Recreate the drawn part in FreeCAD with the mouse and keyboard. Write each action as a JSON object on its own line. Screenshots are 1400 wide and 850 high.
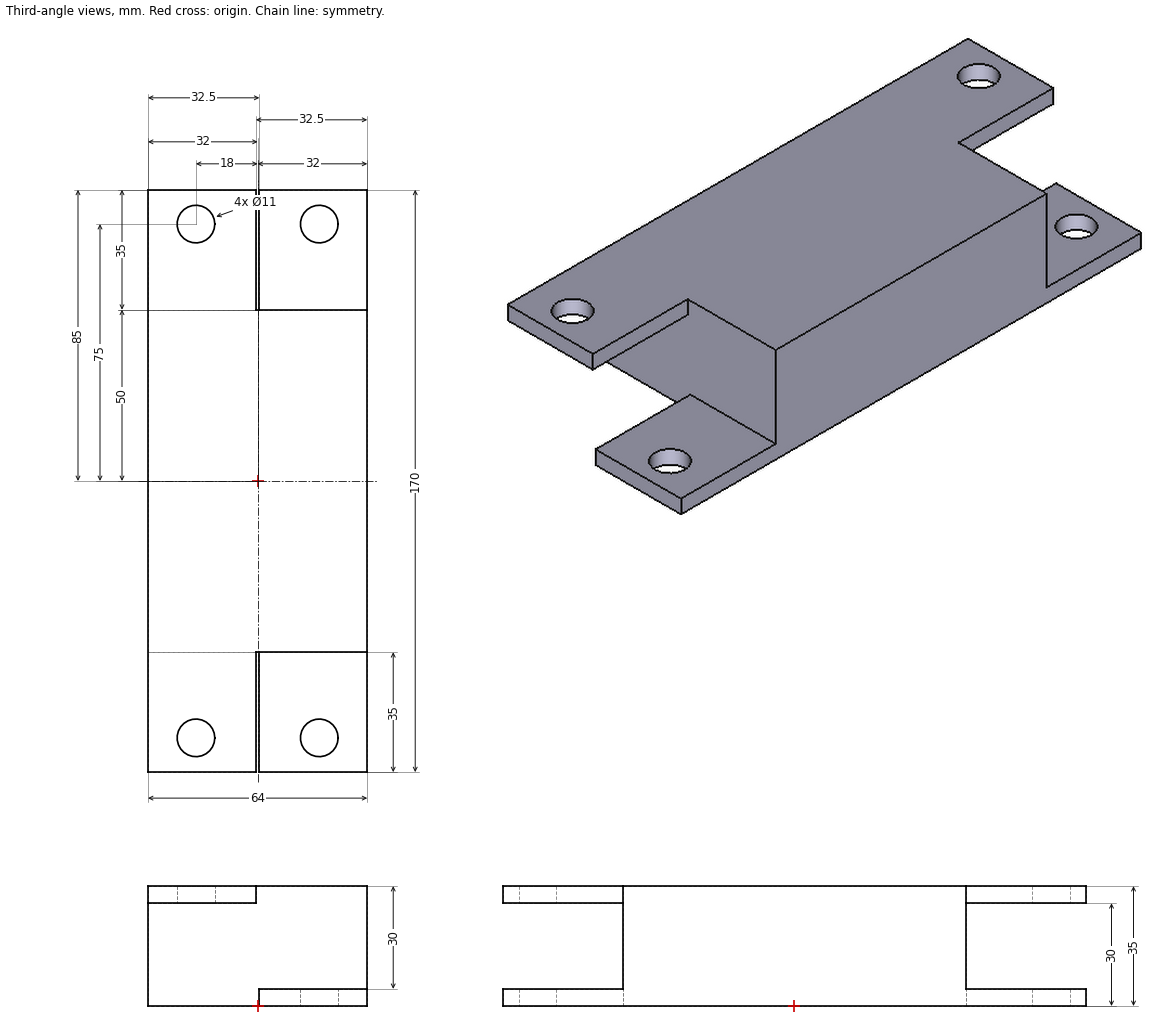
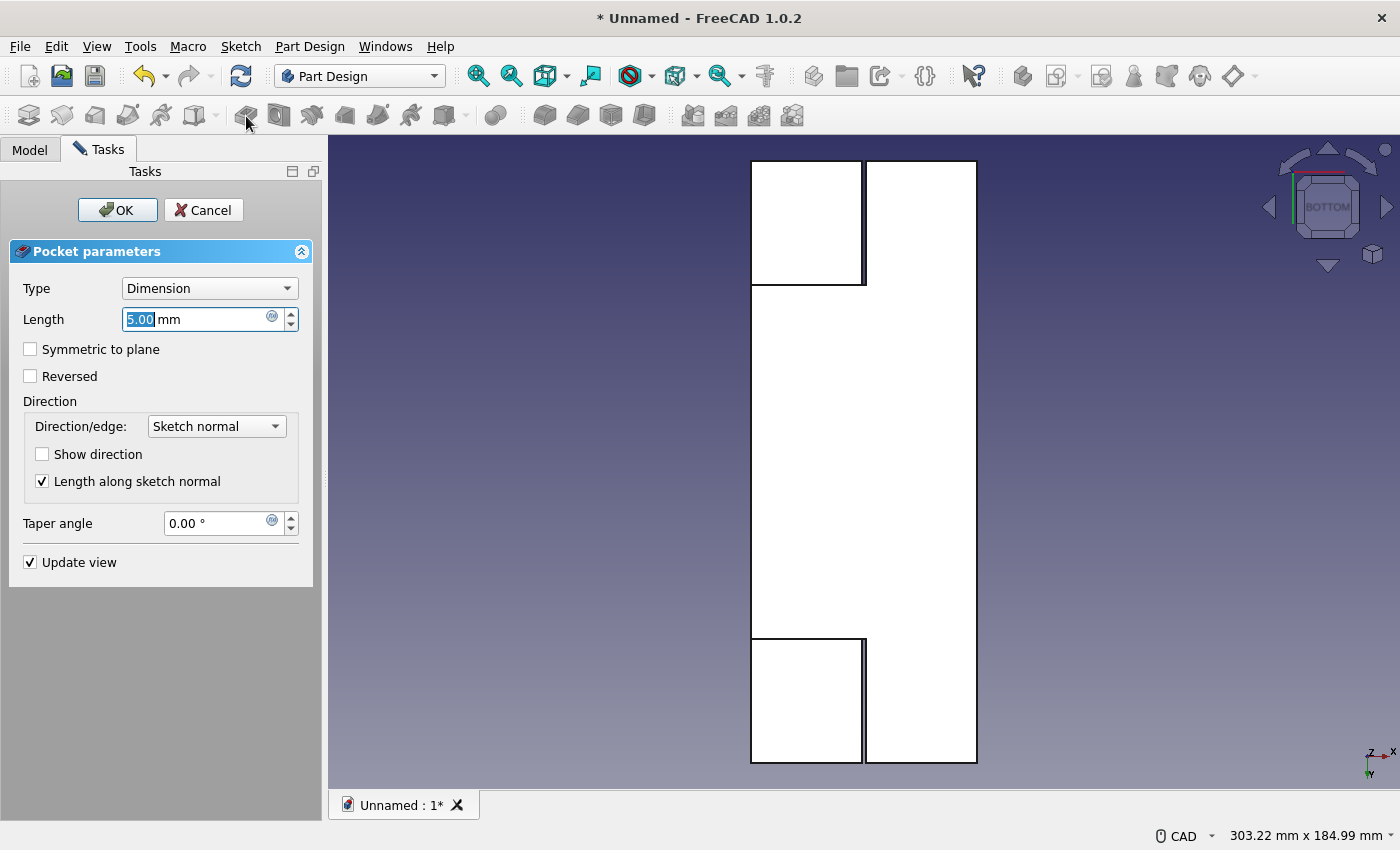
{"action": "type", "text": "30"}
{"action": "key", "text": "Tab"}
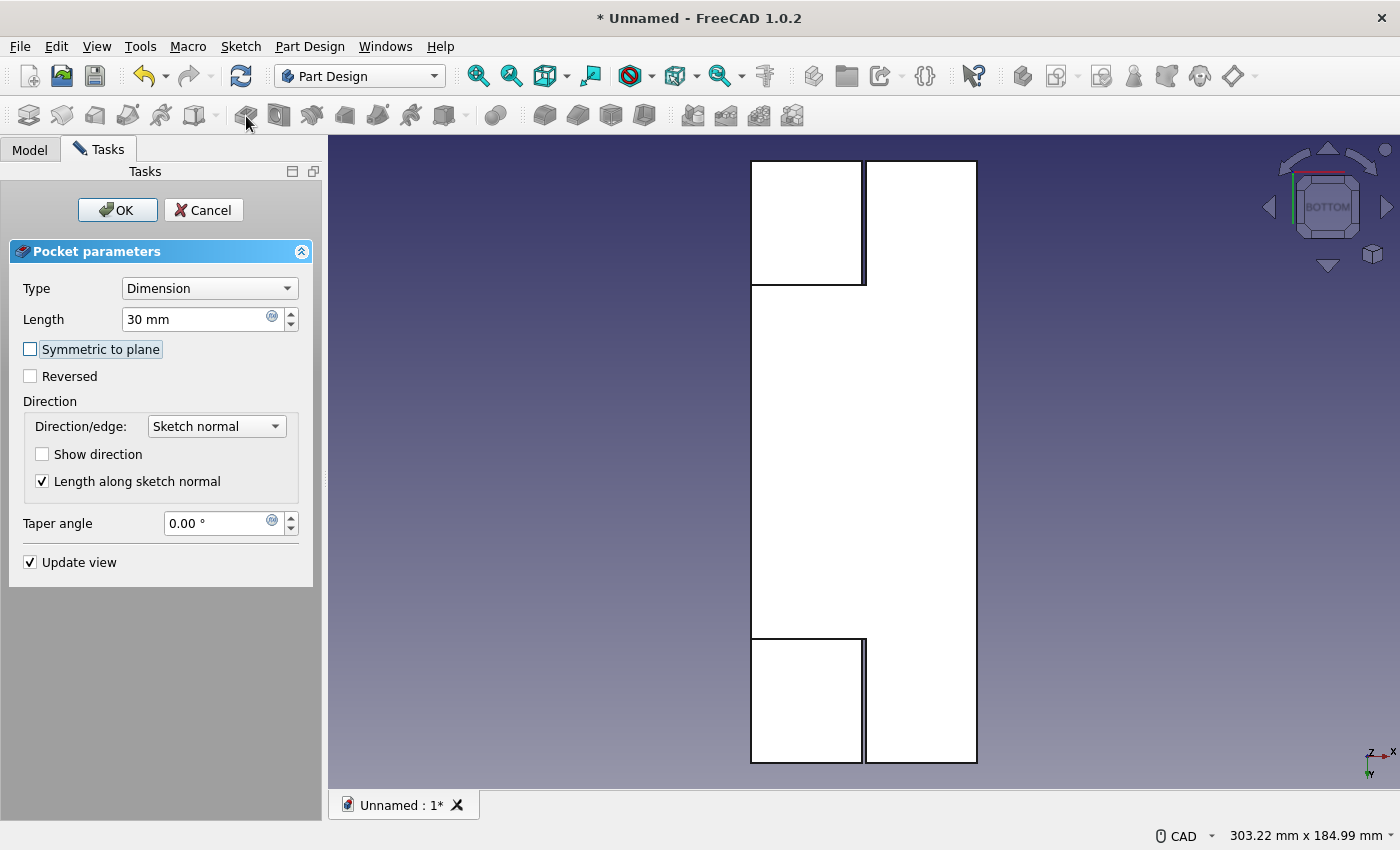
{"action": "left_click", "coordinate": [118, 210]}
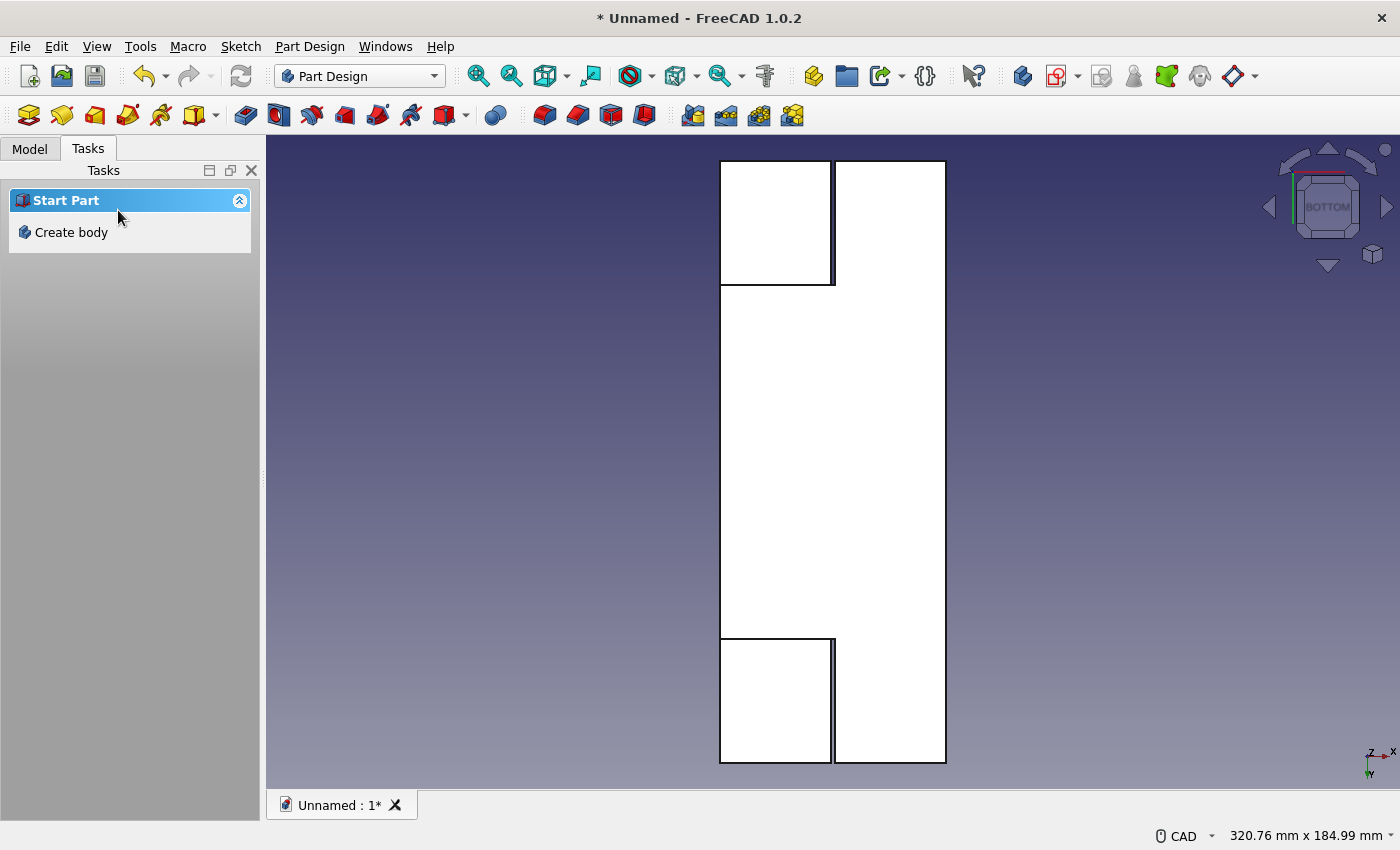
{"action": "key", "text": "0"}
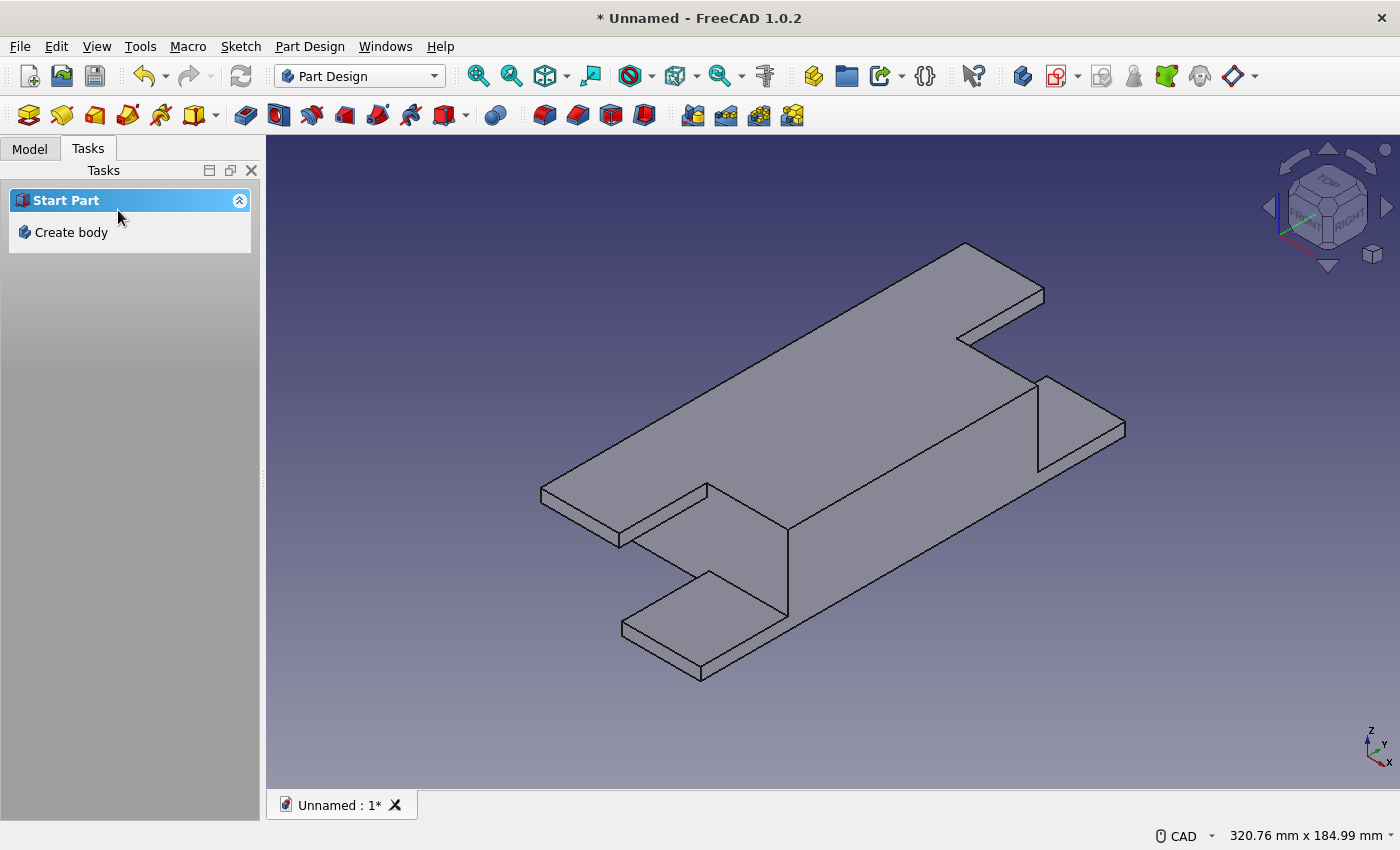
{"action": "left_click", "coordinate": [833, 410]}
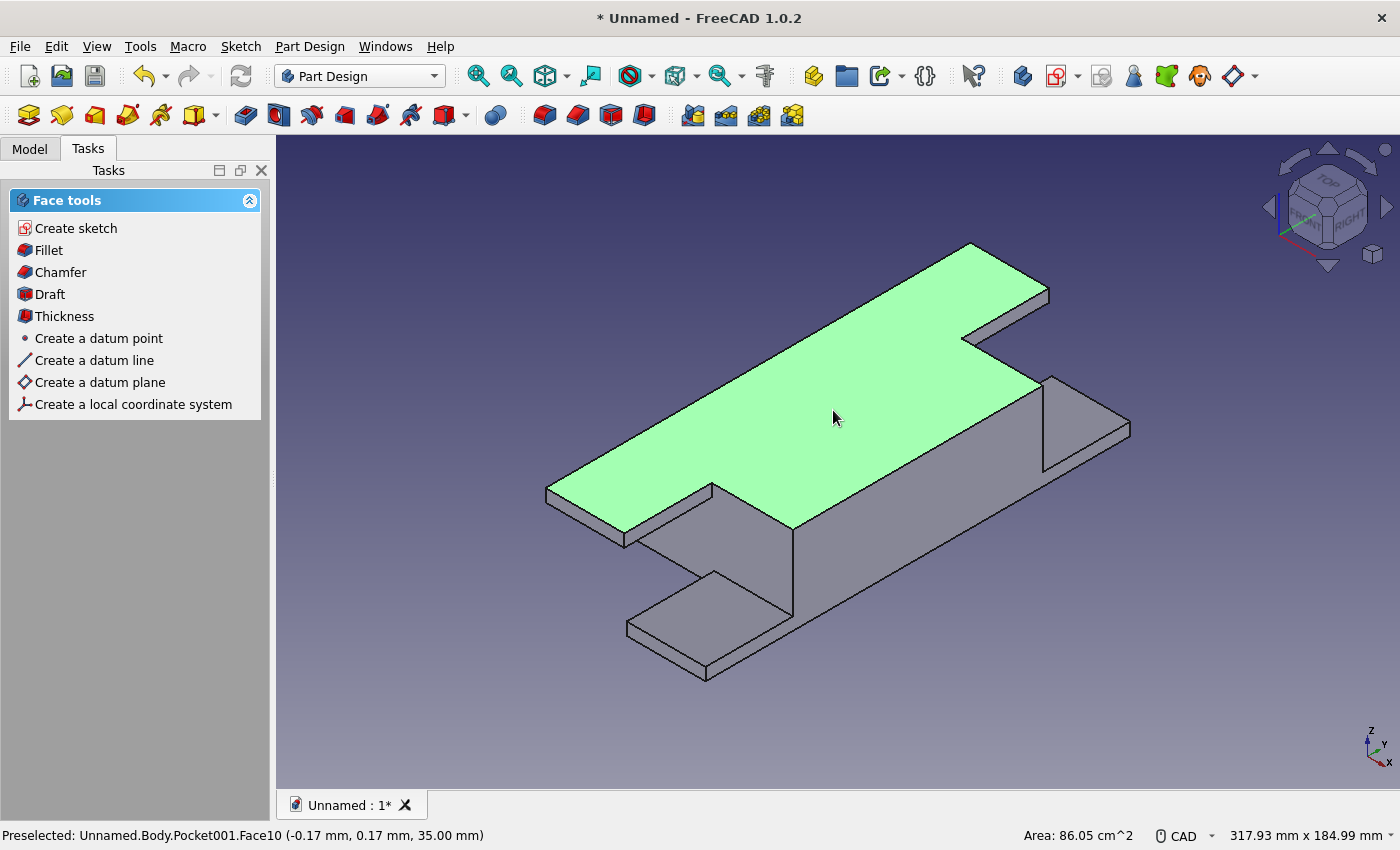
{"action": "left_click", "coordinate": [1056, 76]}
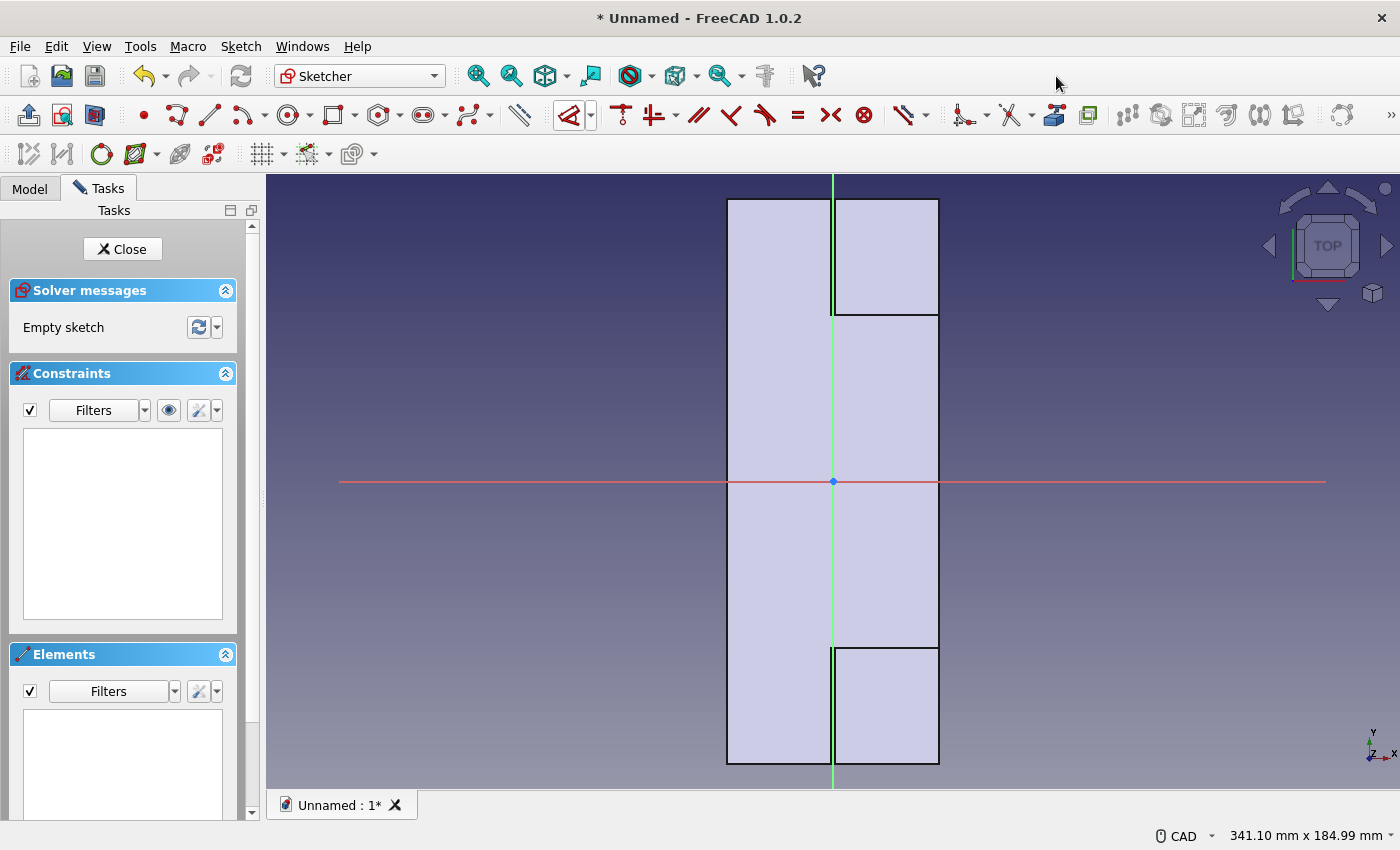
{"action": "scroll", "coordinate": [625, 482], "scroll_direction": "down", "scroll_amount": 2}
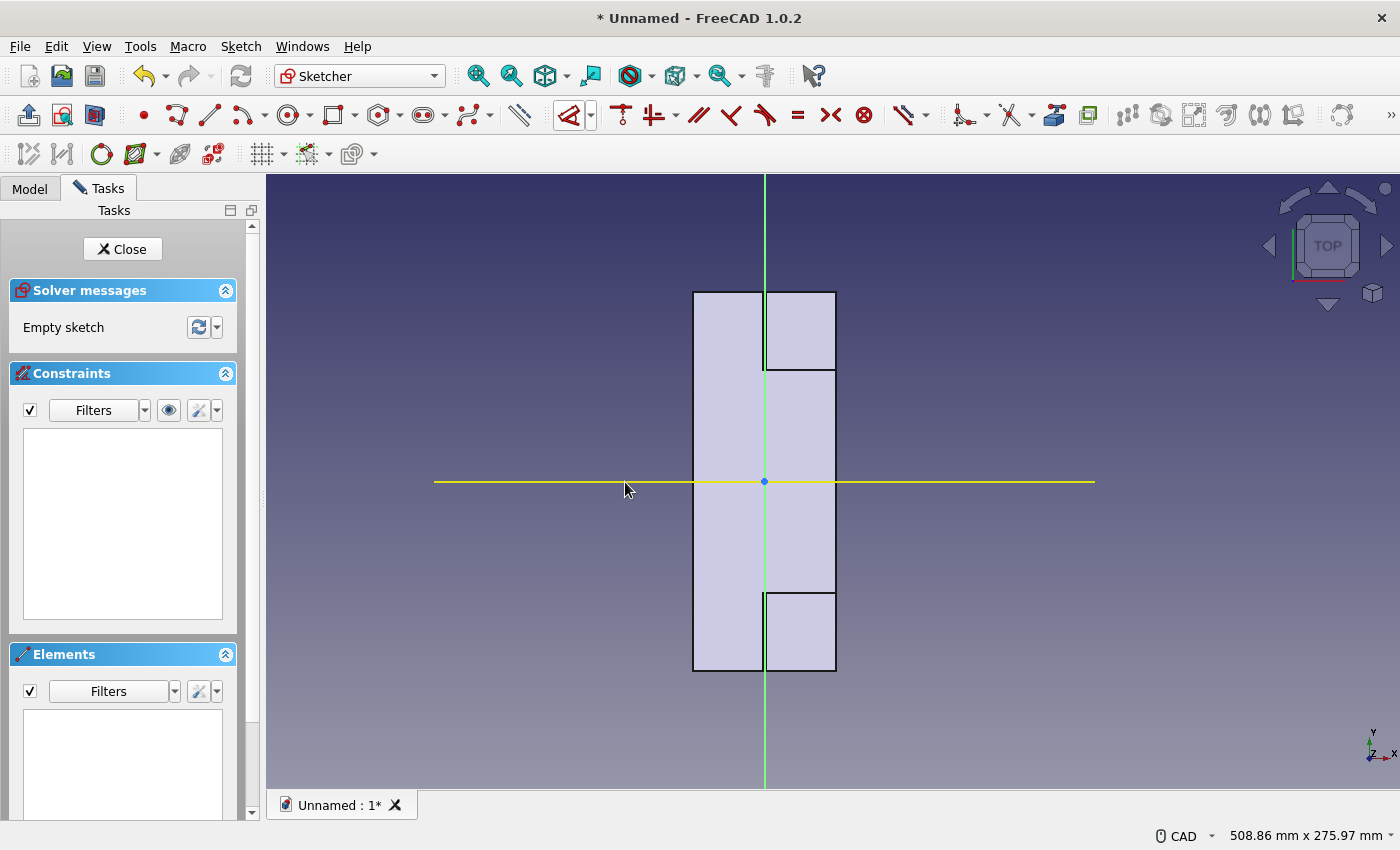
{"action": "left_click", "coordinate": [288, 116]}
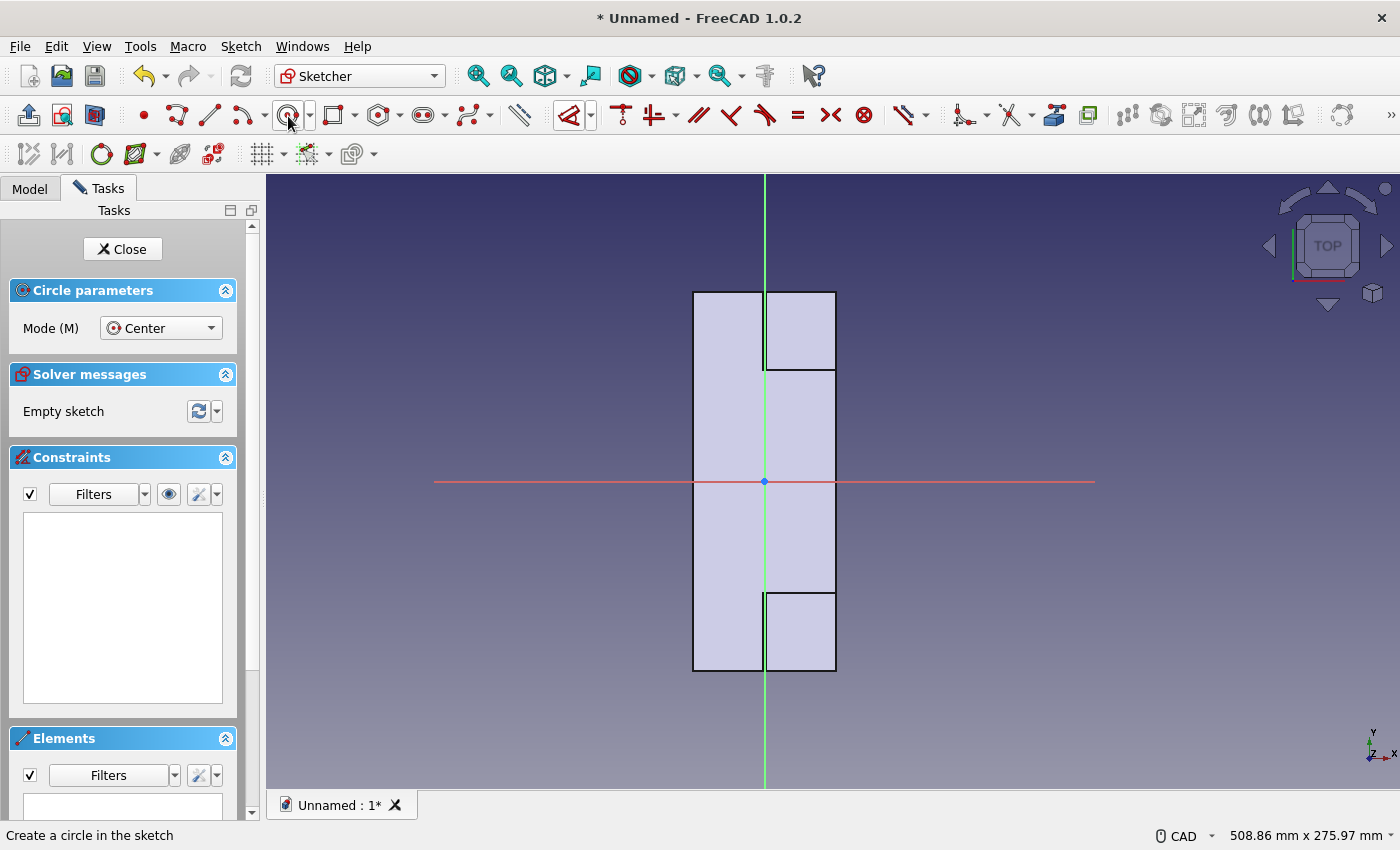
{"action": "scroll", "coordinate": [724, 315], "scroll_direction": "up", "scroll_amount": 4}